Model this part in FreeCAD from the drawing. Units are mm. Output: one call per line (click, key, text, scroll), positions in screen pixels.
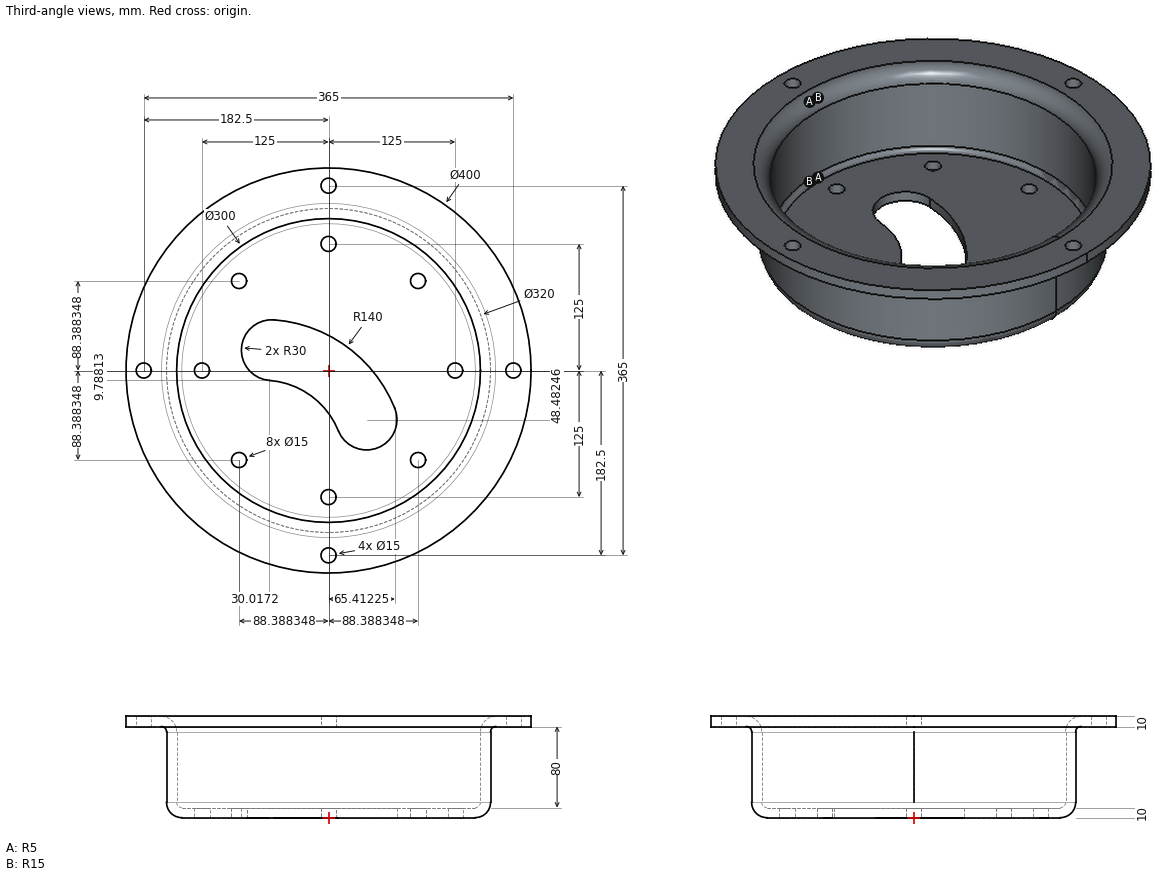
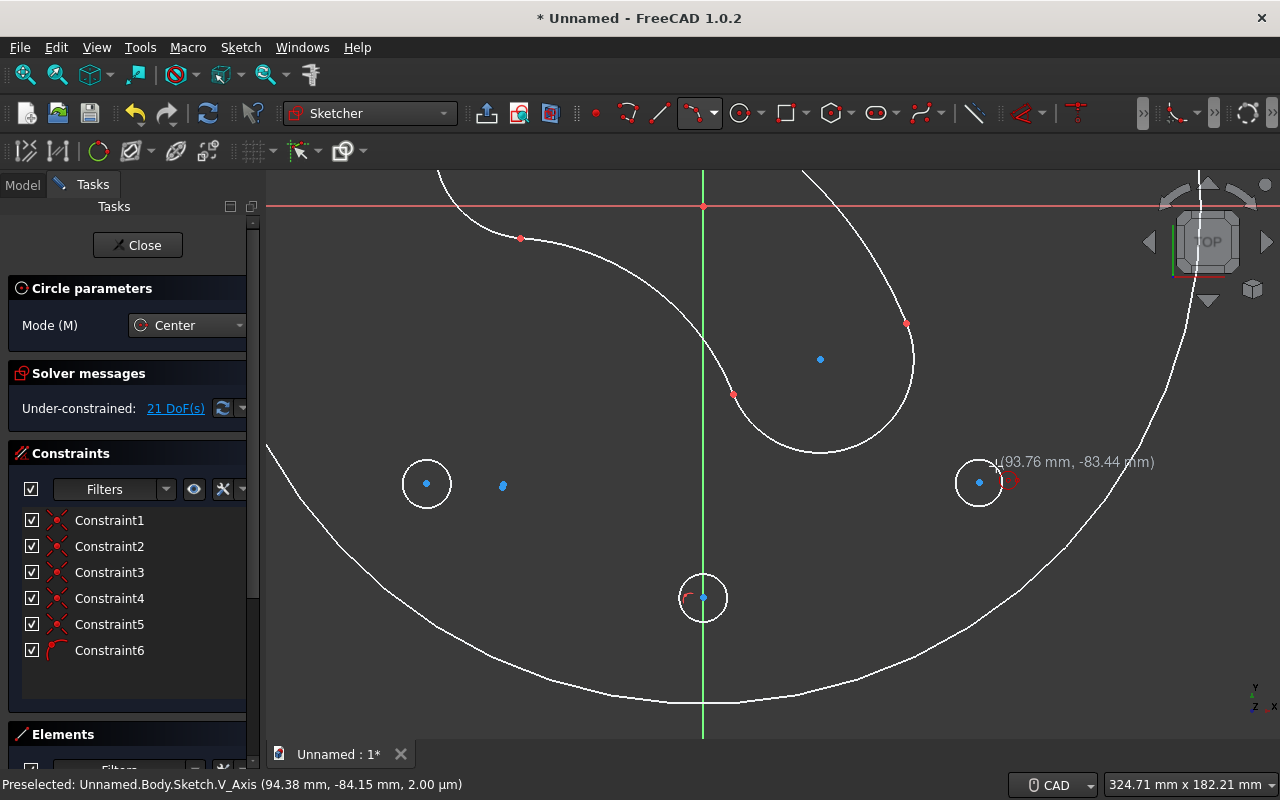
click(313, 206)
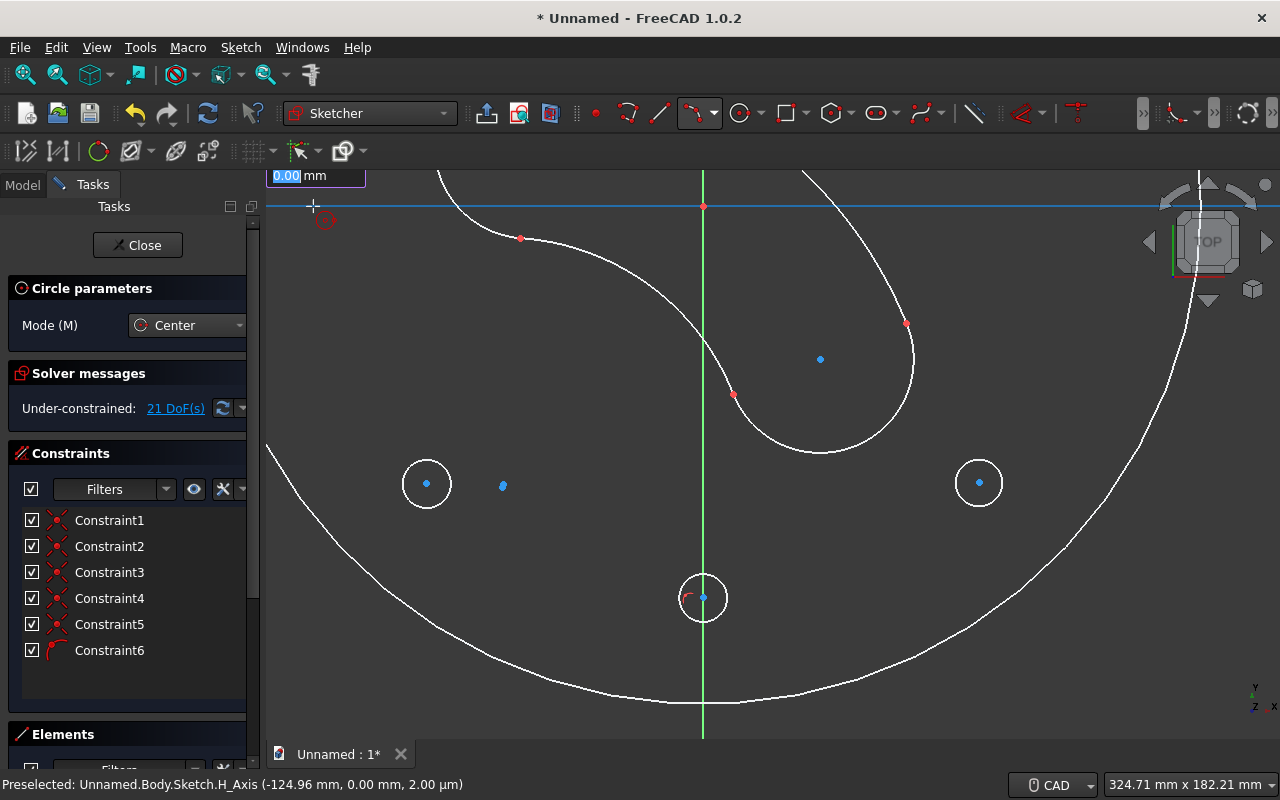
scroll(705, 599, down, 5)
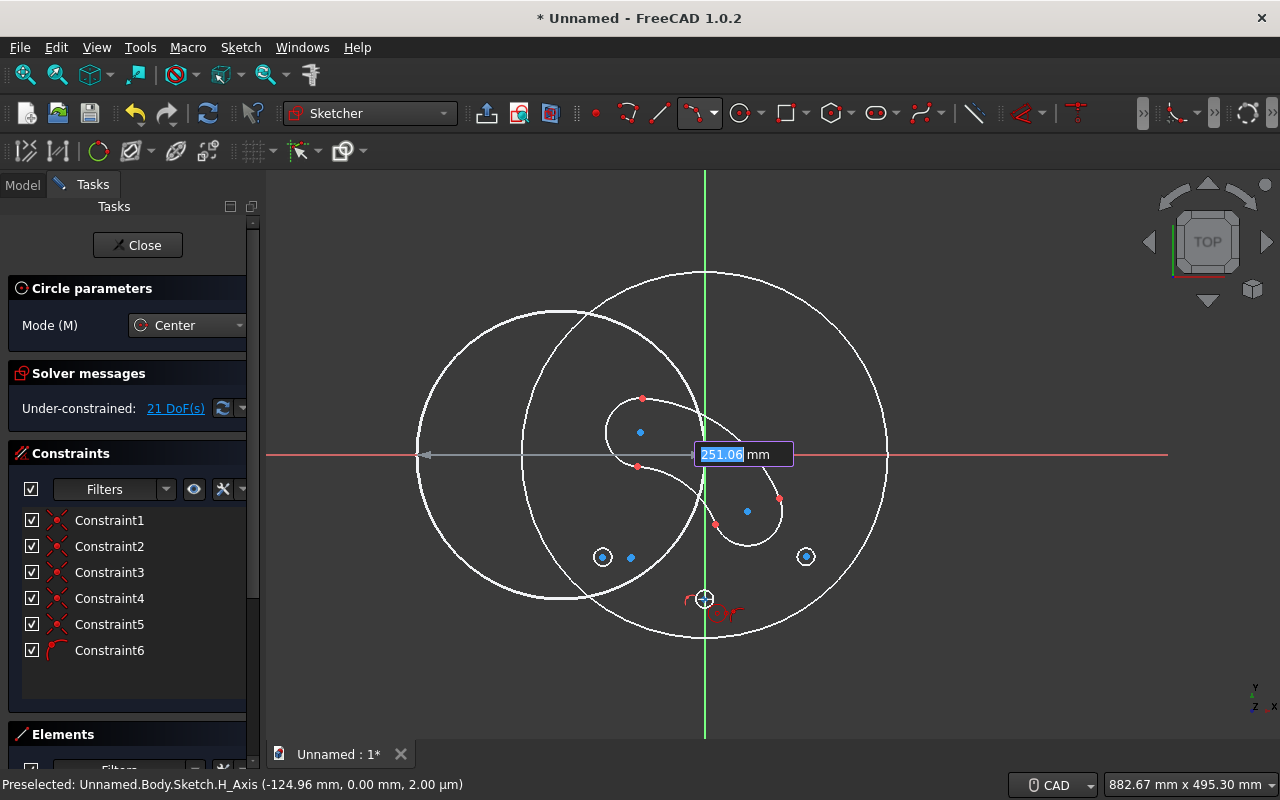
scroll(567, 449, up, 5)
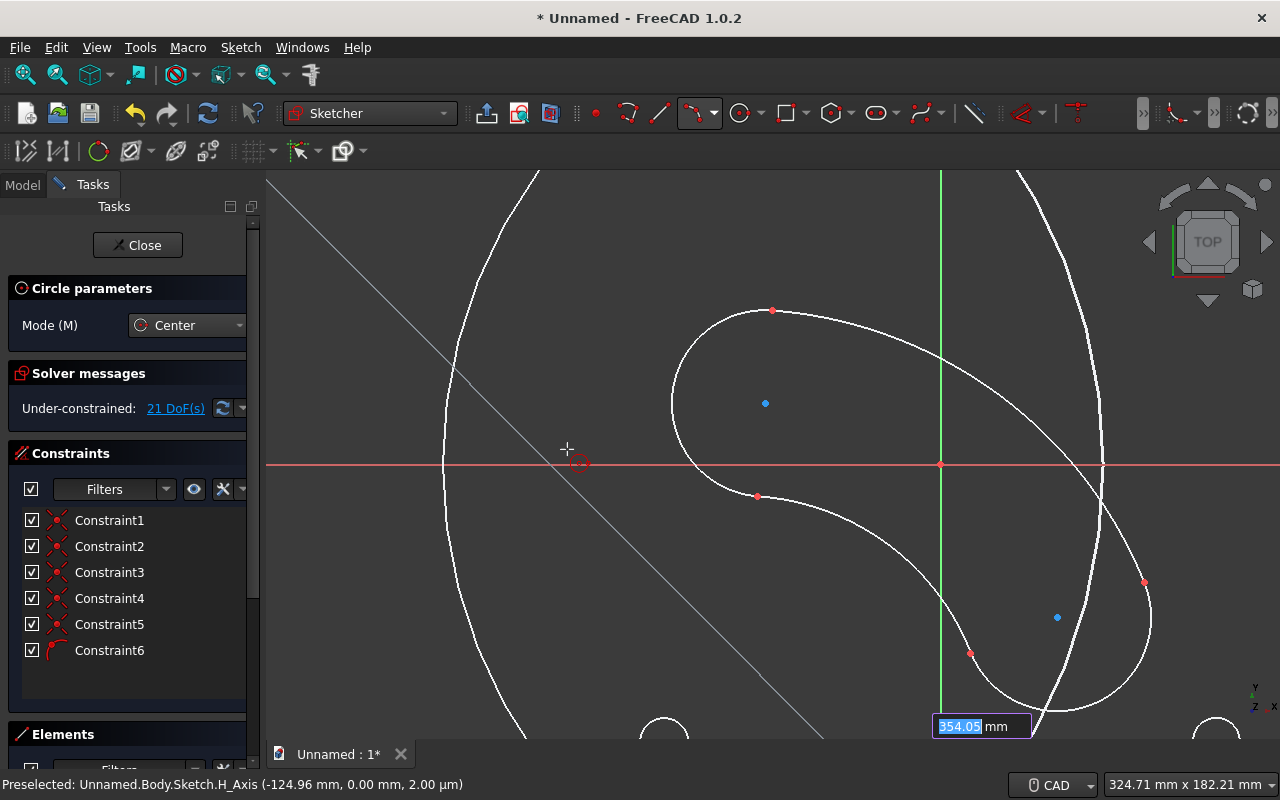
click(567, 448)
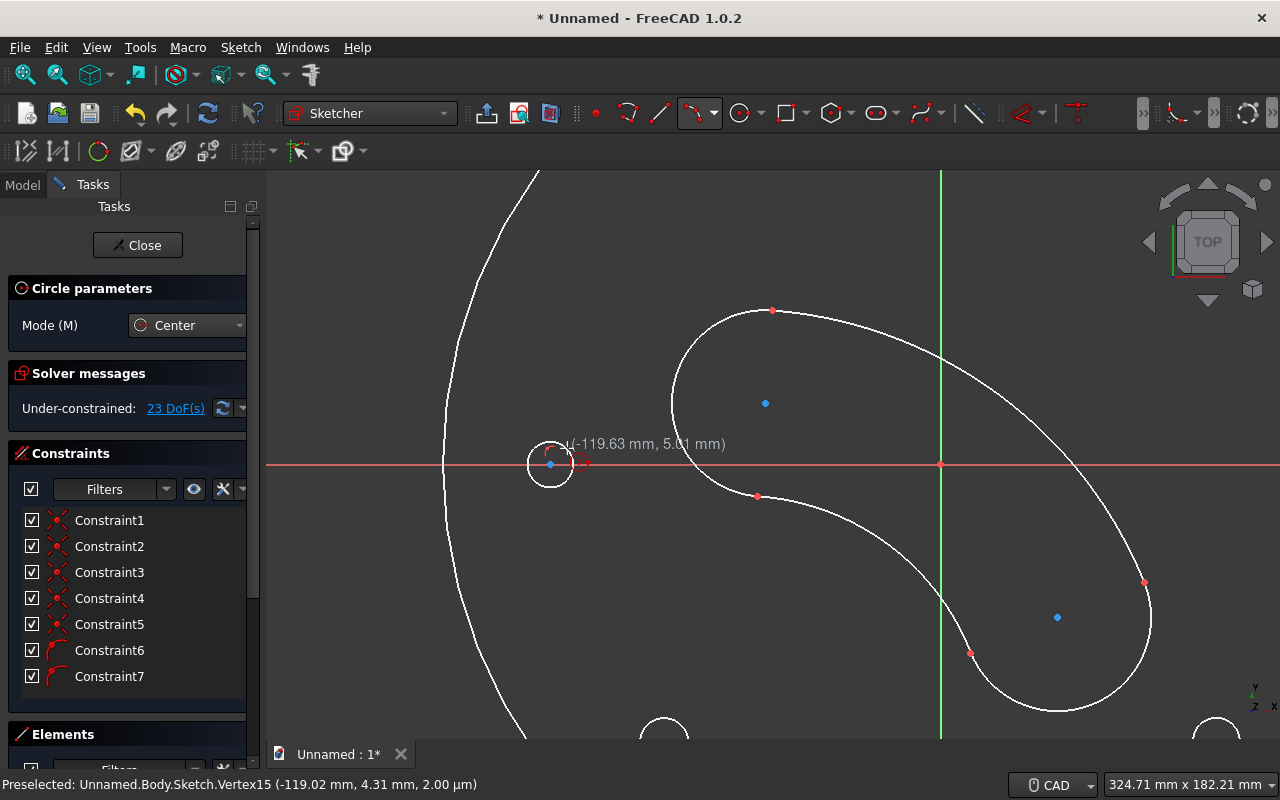
scroll(567, 449, down, 5)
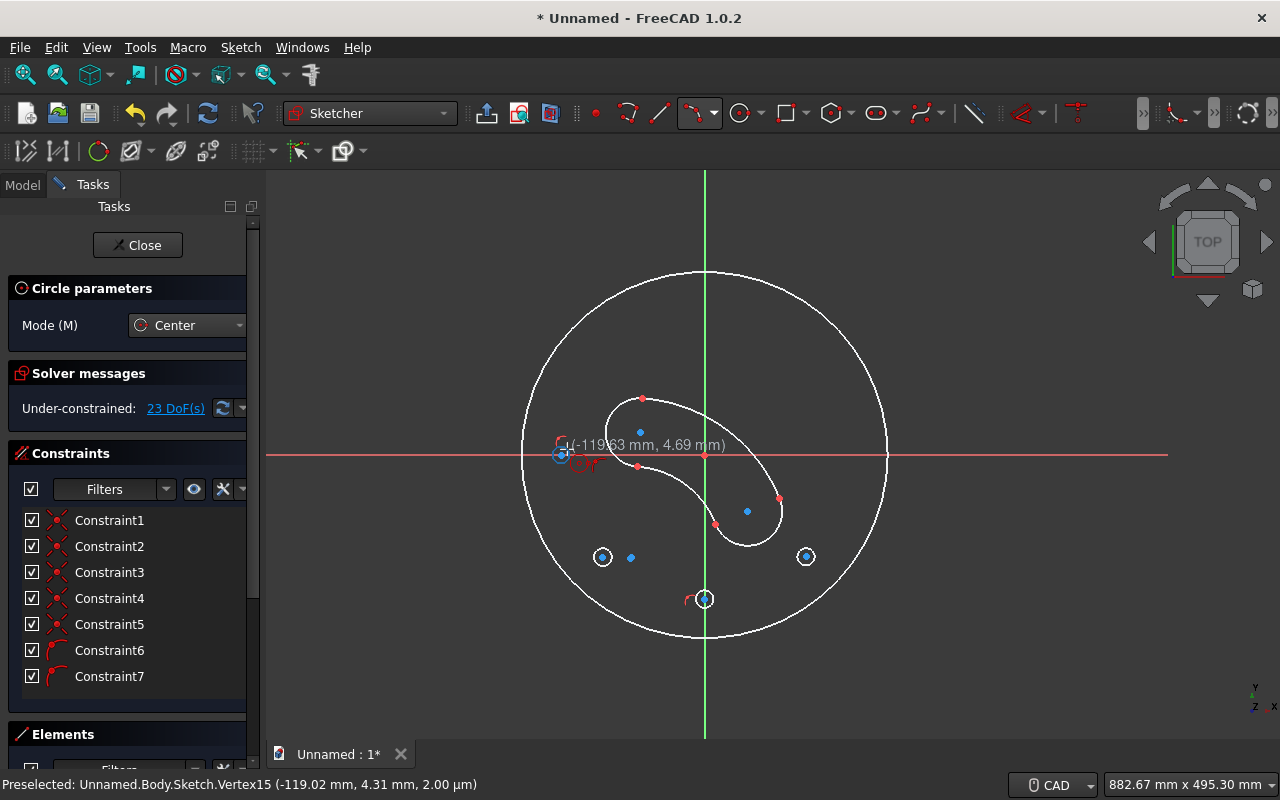
scroll(603, 354, up, 5)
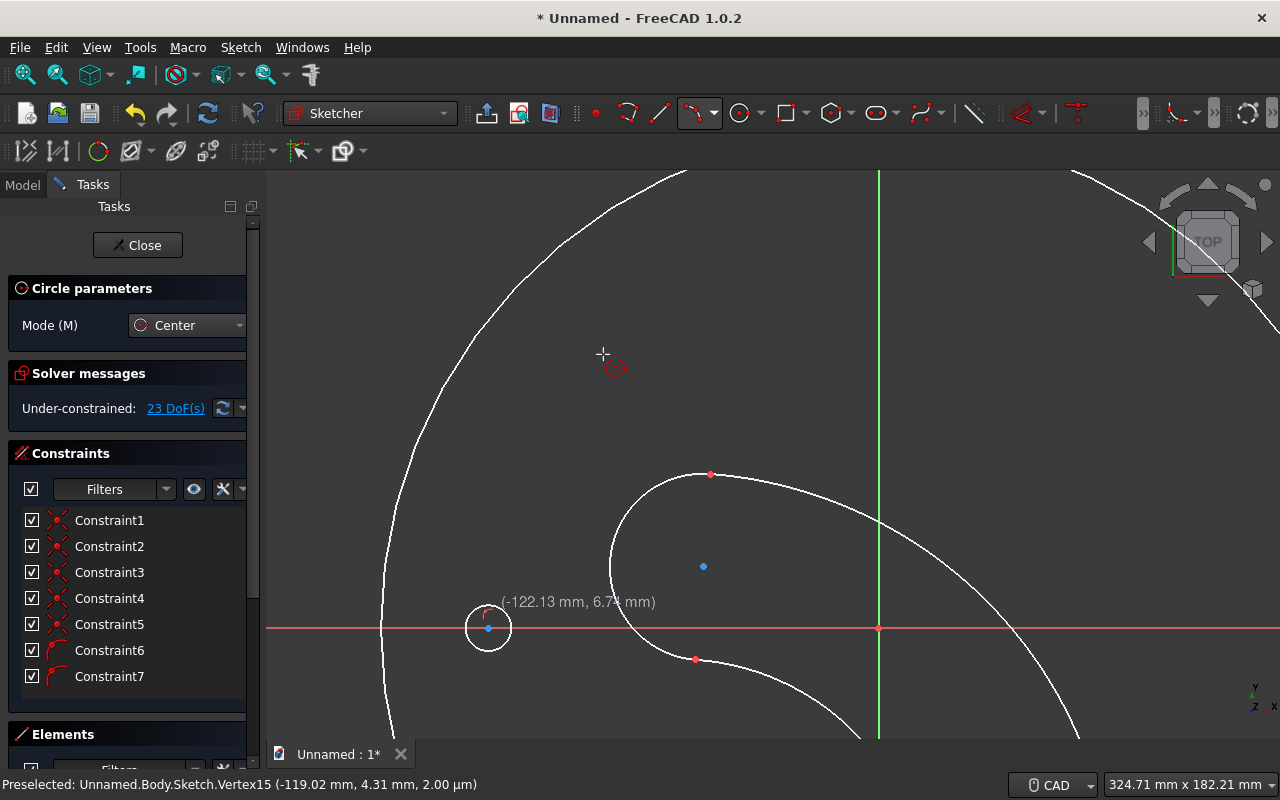
click(603, 352)
click(619, 336)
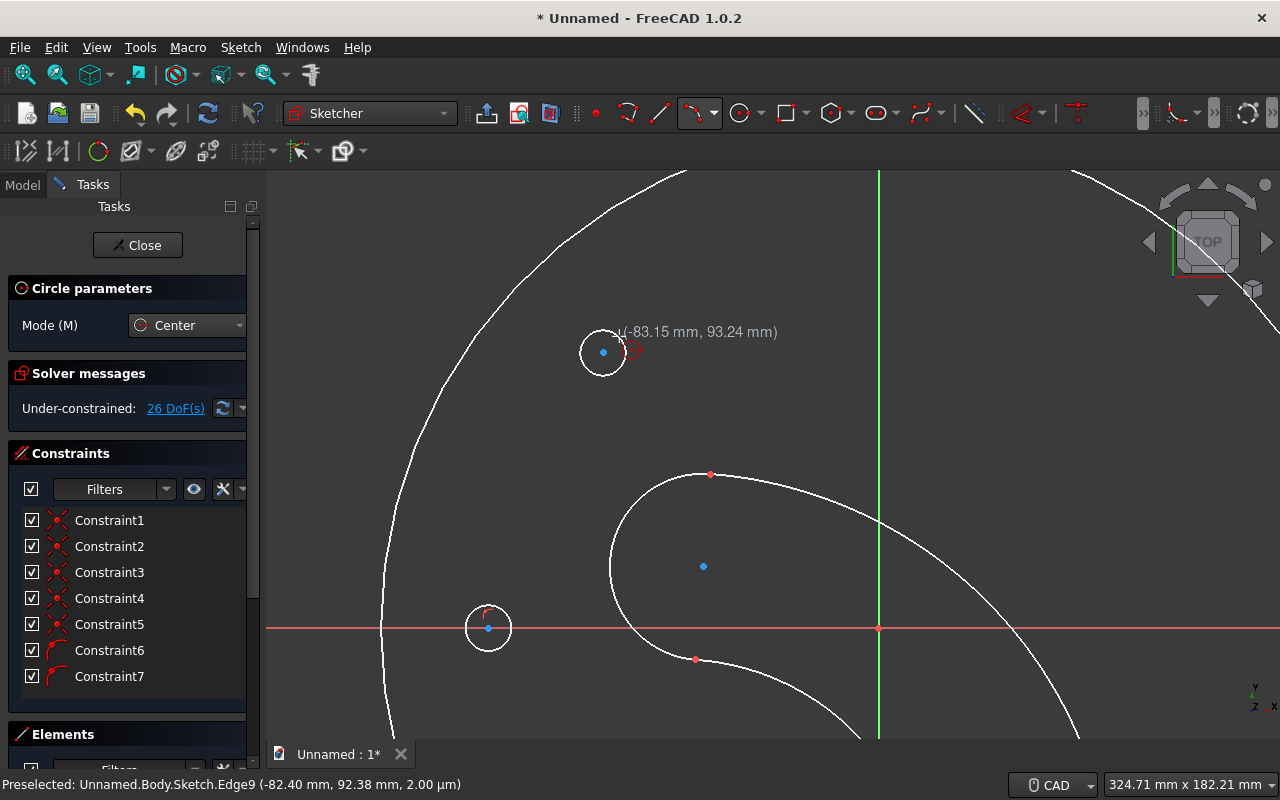
scroll(603, 353, down, 5)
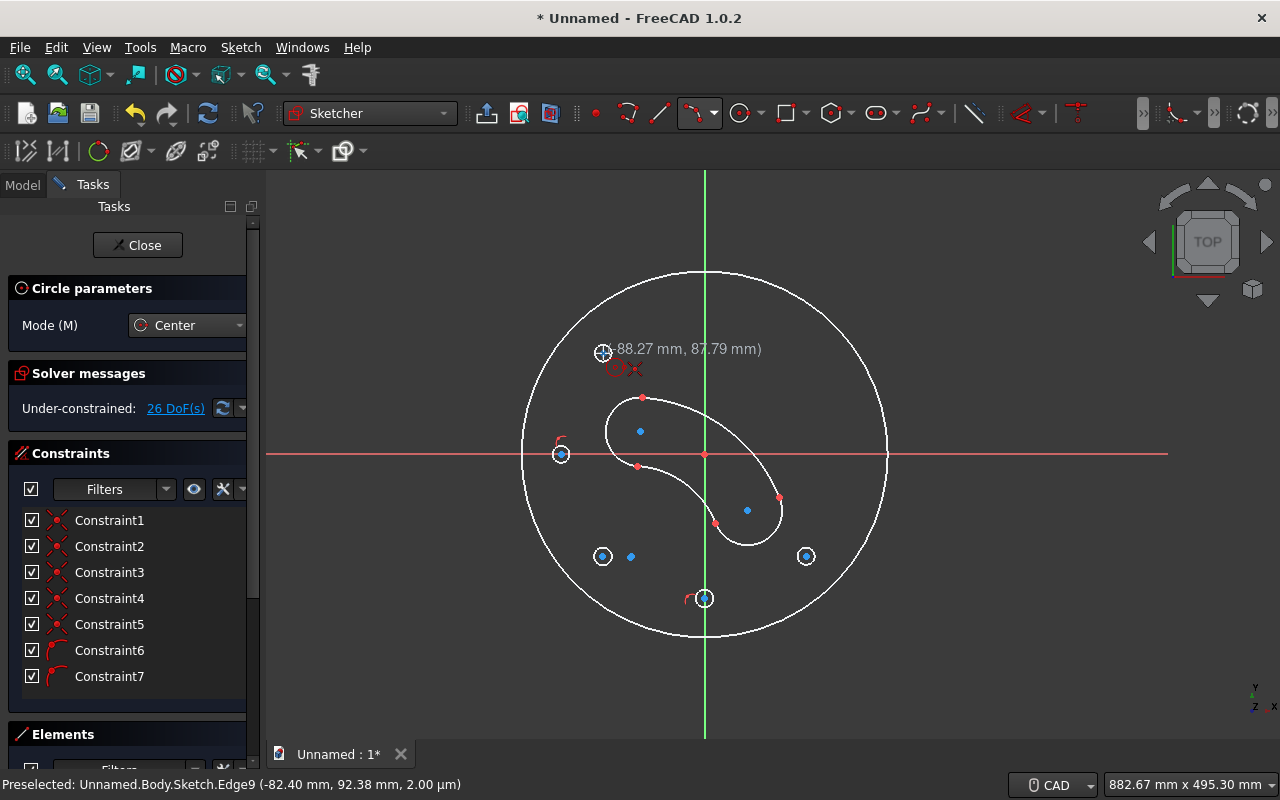
scroll(848, 454, up, 5)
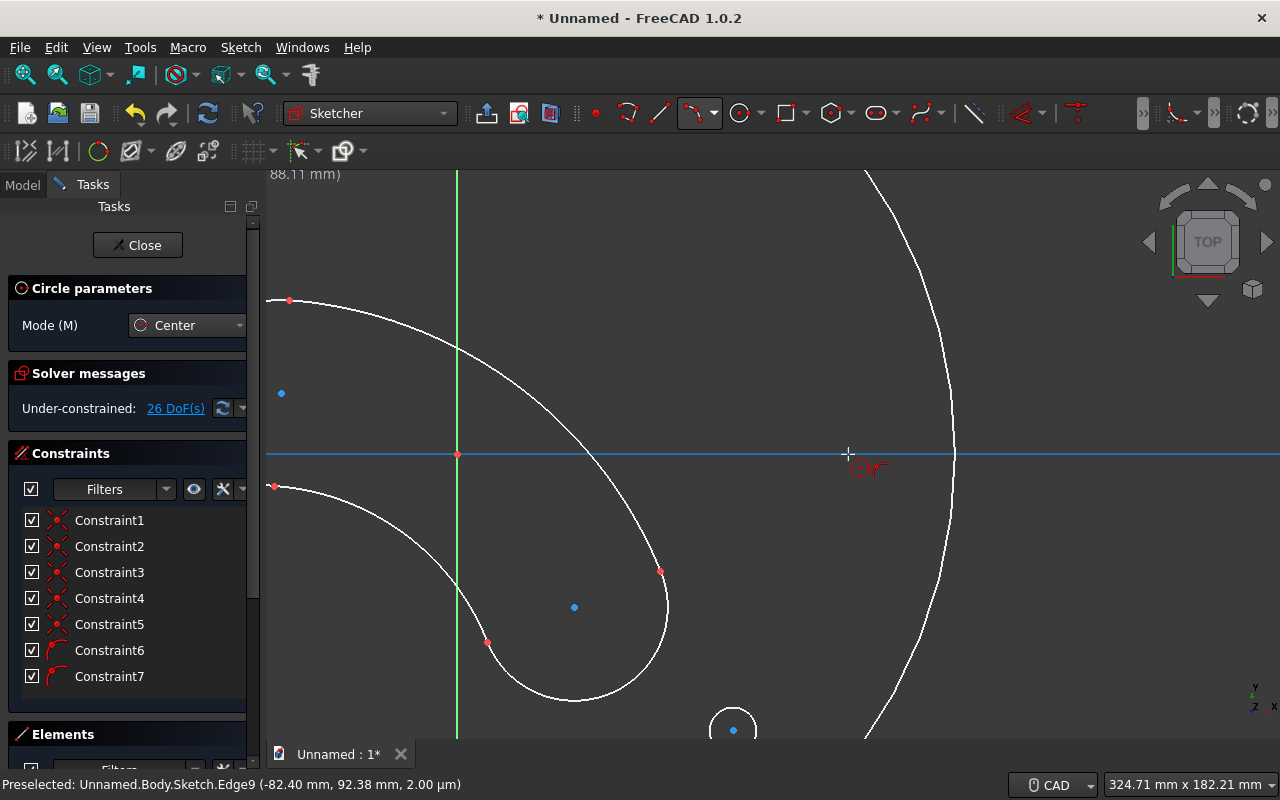
click(848, 454)
click(864, 438)